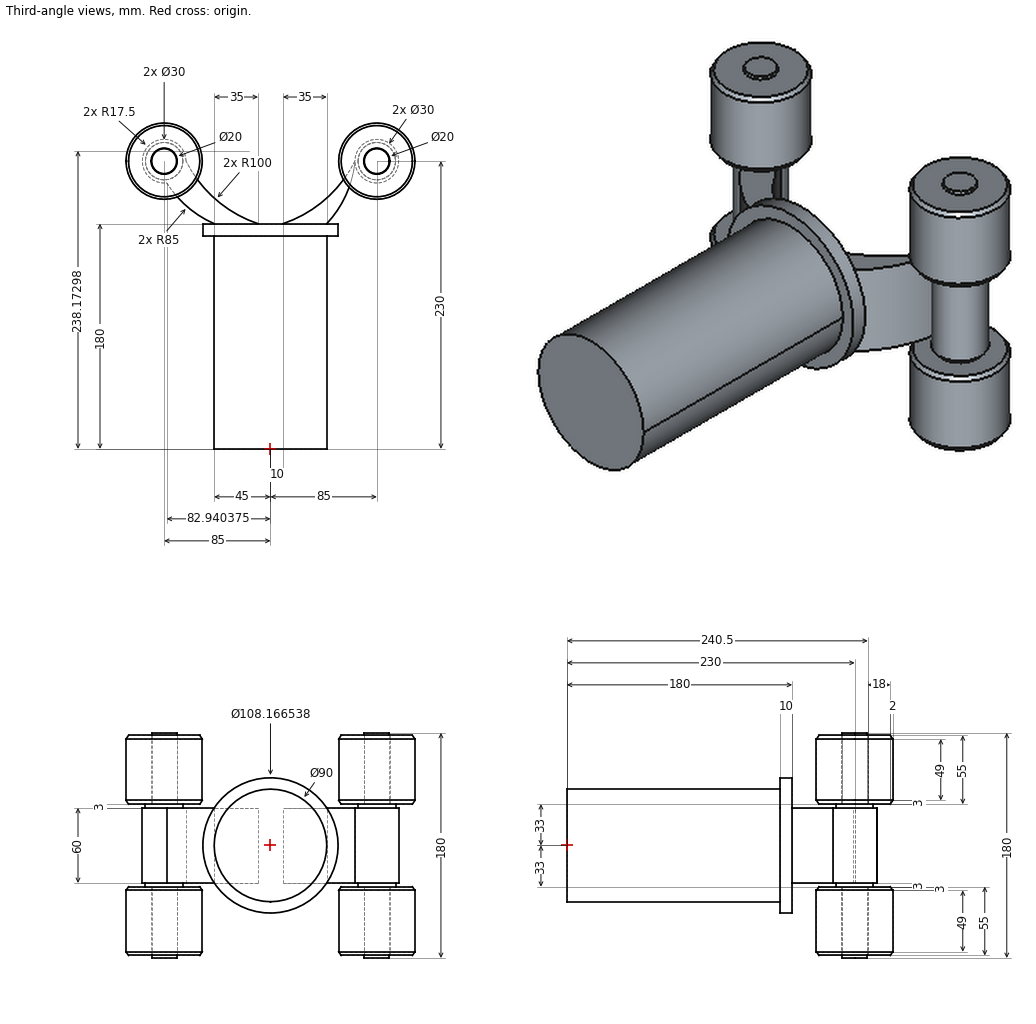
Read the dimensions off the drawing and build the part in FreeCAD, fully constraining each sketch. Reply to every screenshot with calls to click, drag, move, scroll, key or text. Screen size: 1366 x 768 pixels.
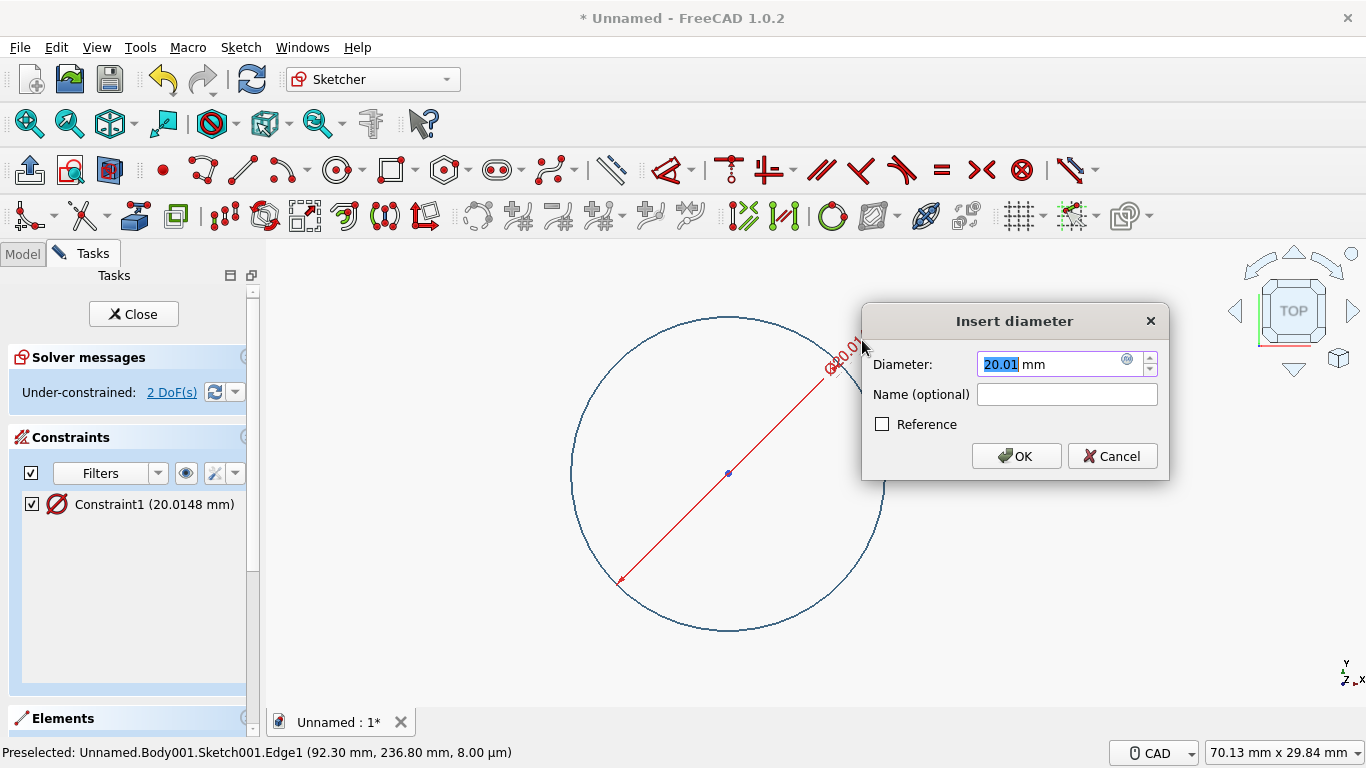
text(20)
key(Return)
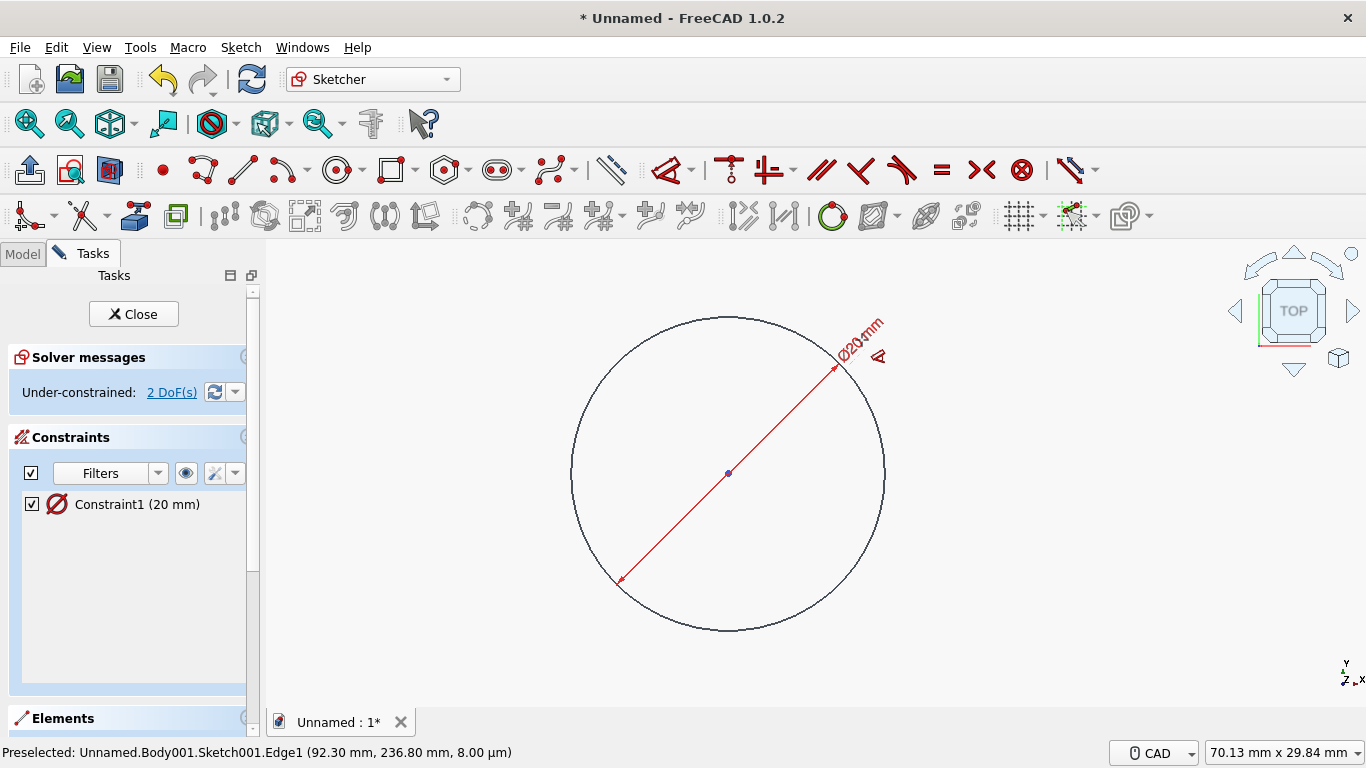
click(728, 474)
click(511, 440)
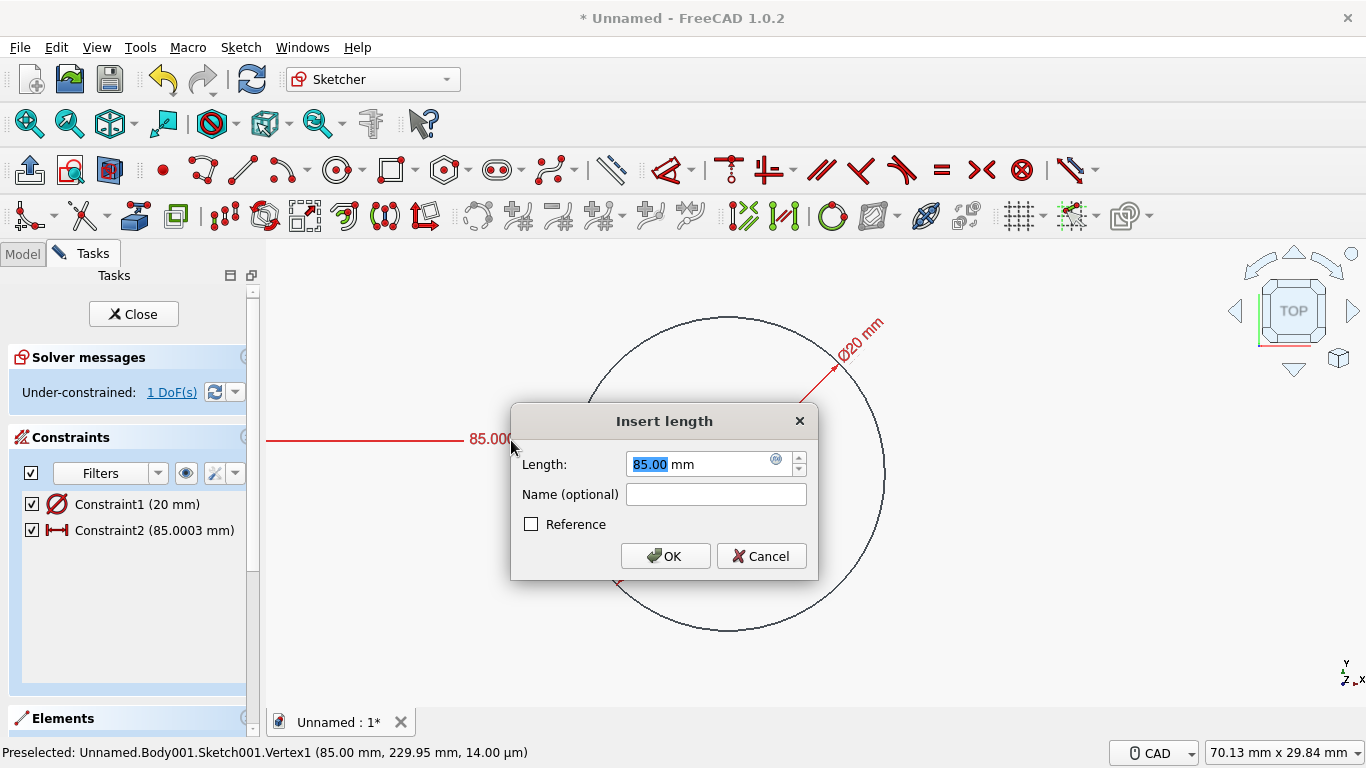
text(85)
key(Return)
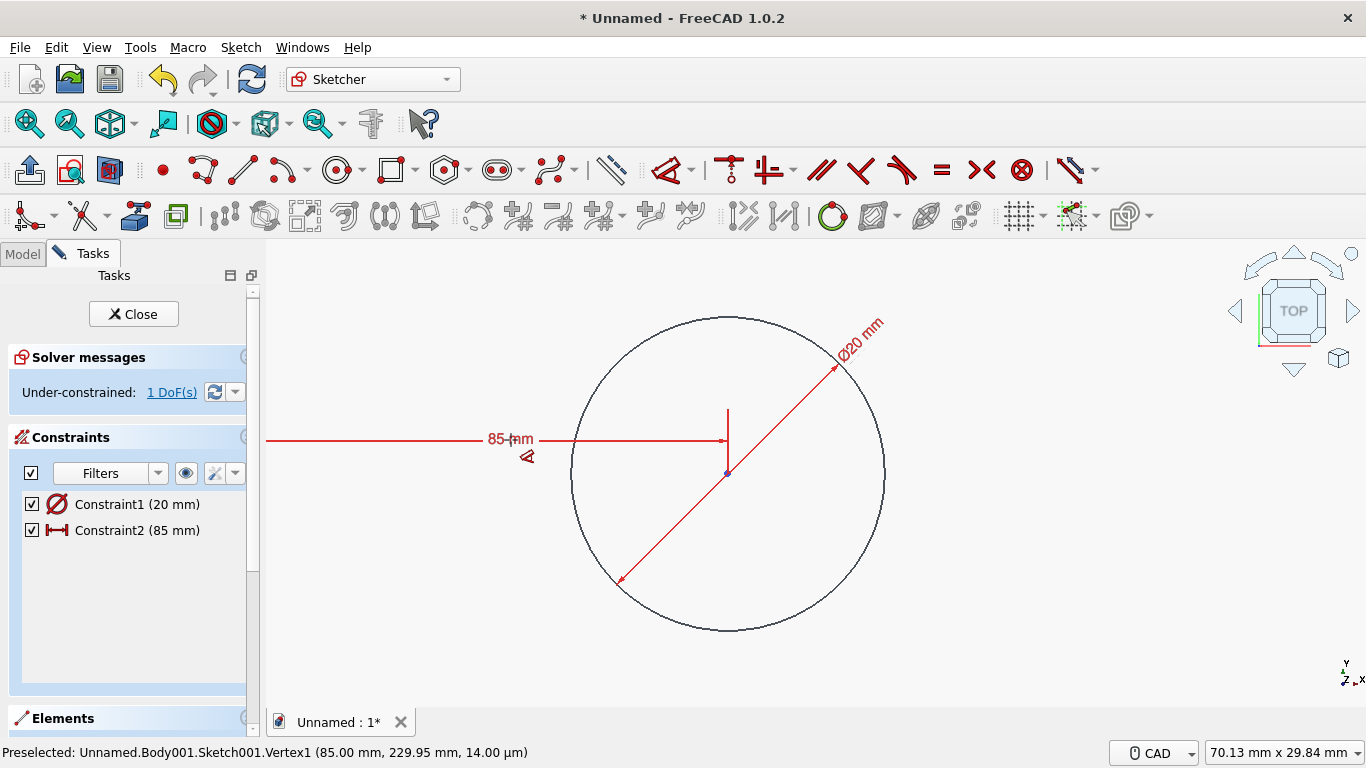
click(728, 474)
click(762, 577)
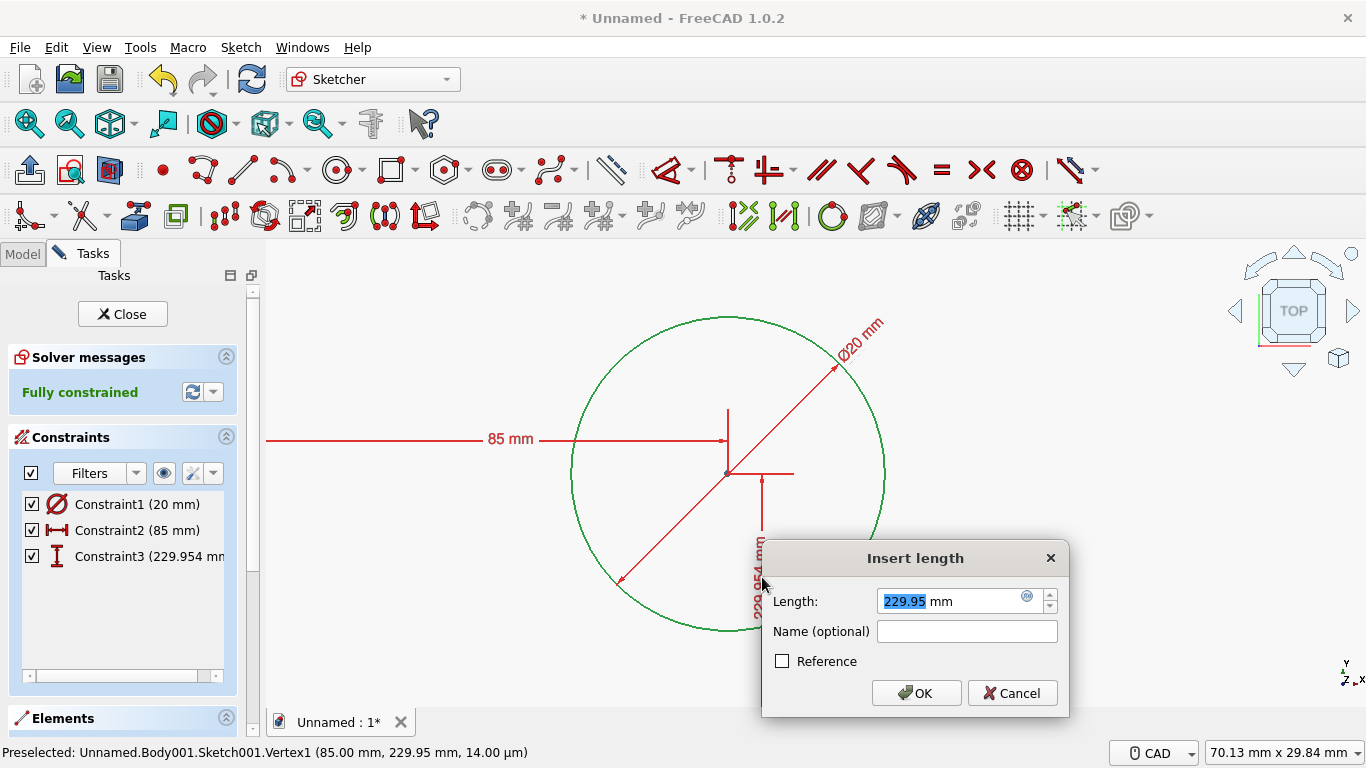
text(230)
key(Return)
key(Escape)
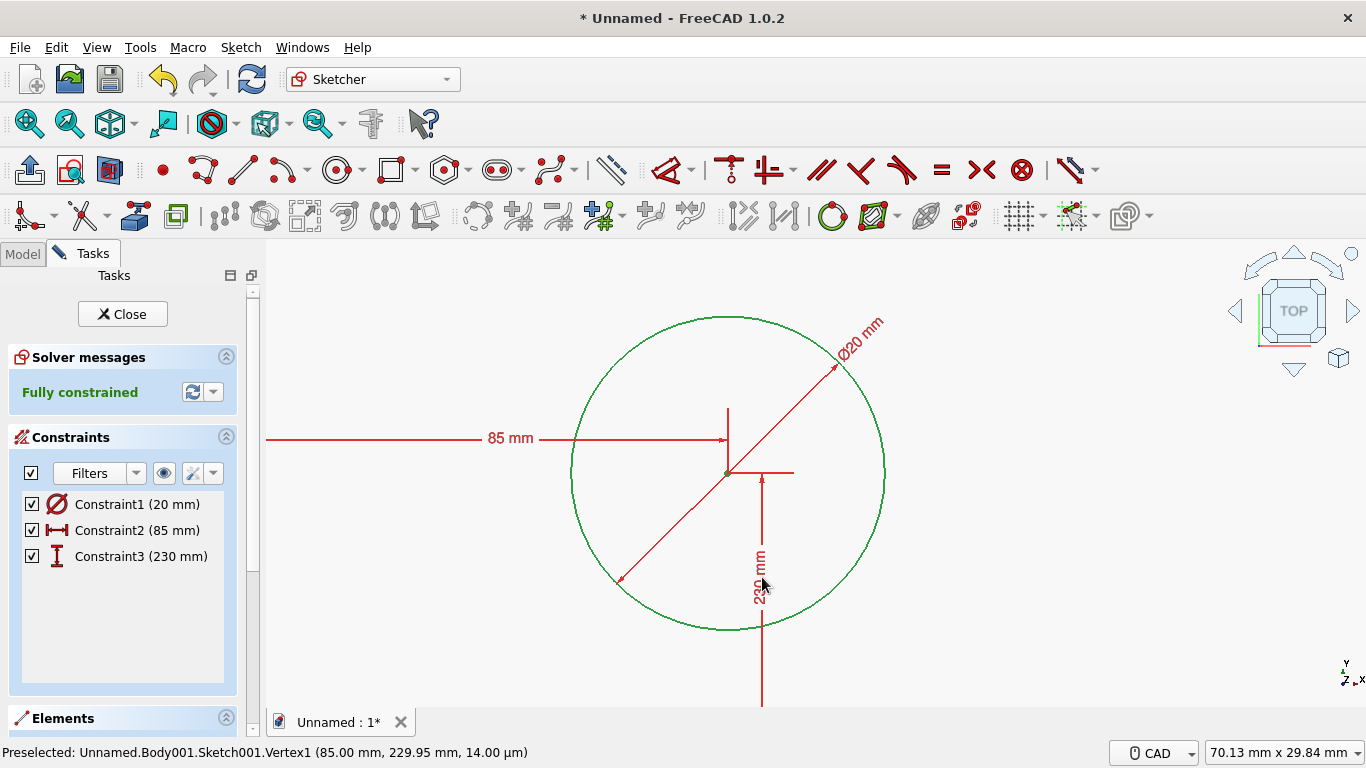
click(123, 314)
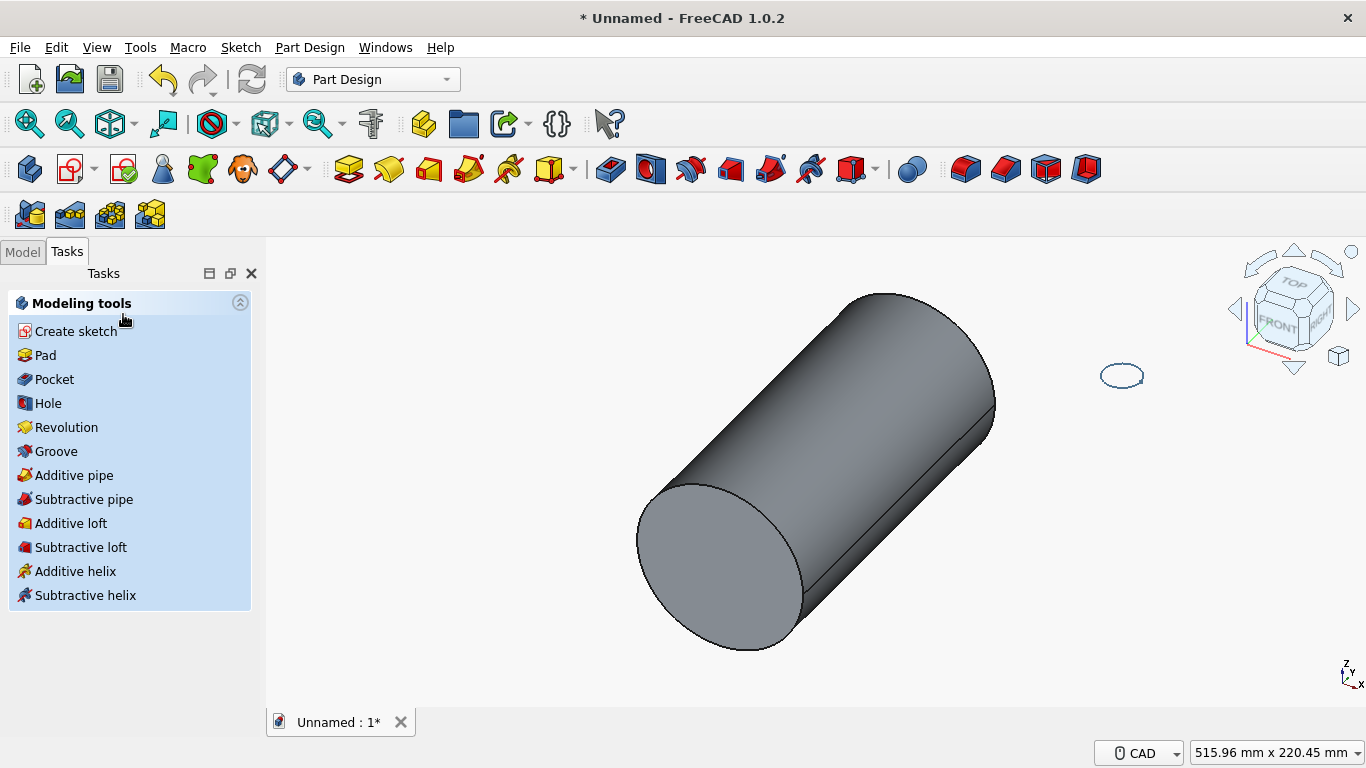
click(350, 170)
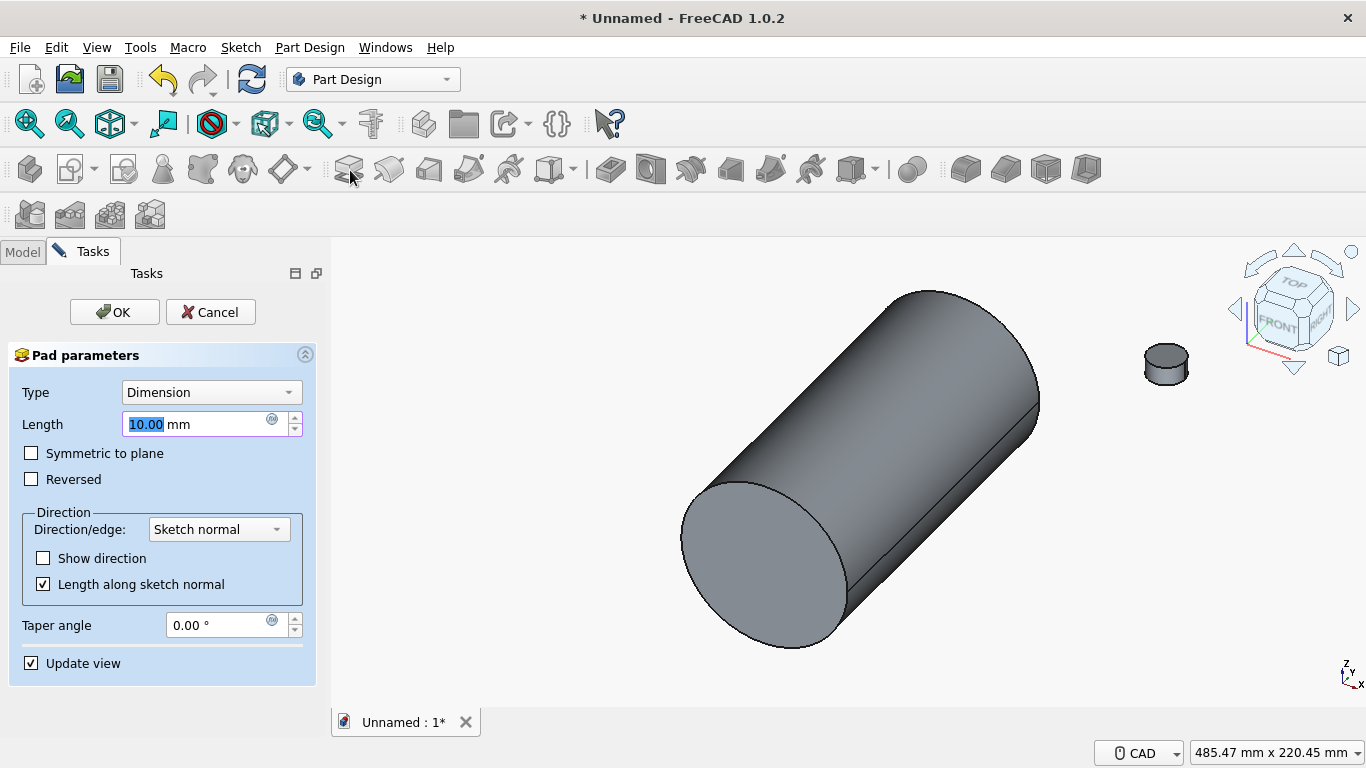
text(180)
key(Tab)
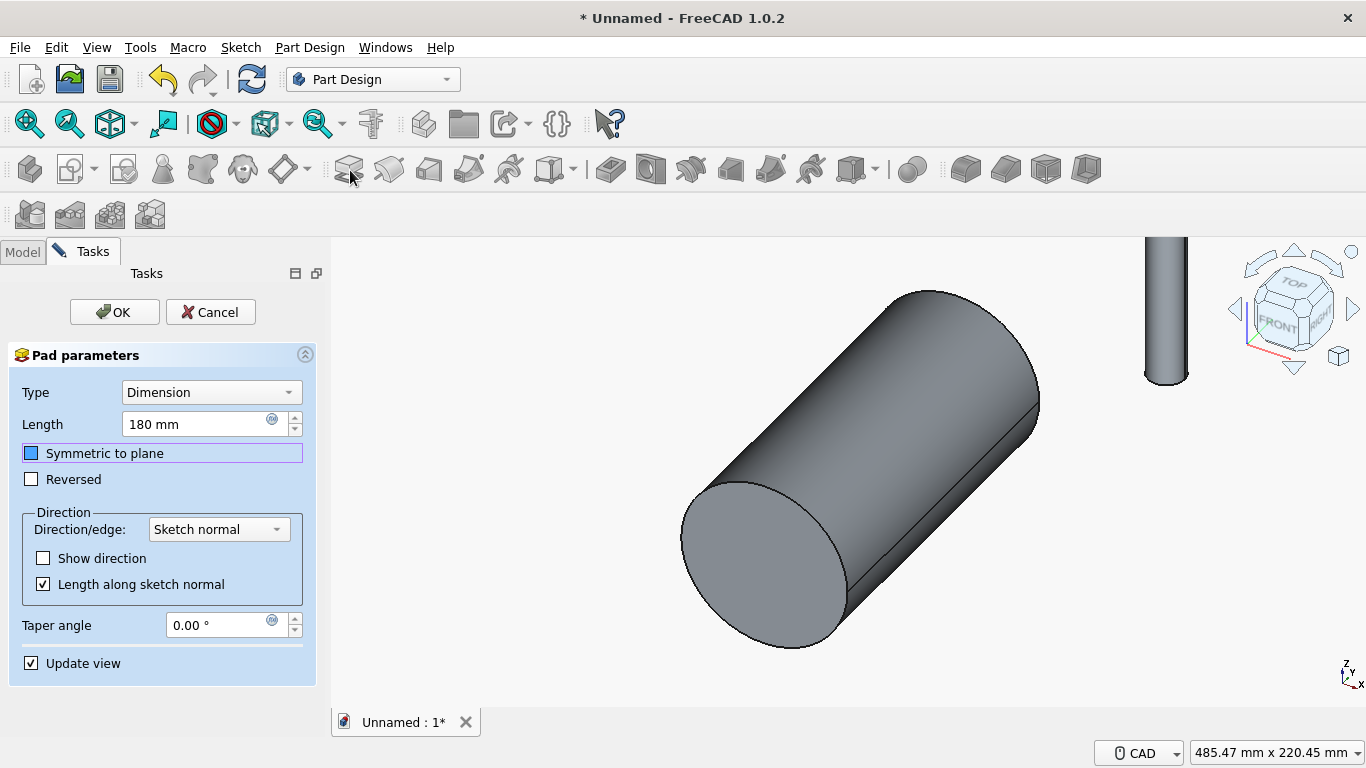
click(30, 453)